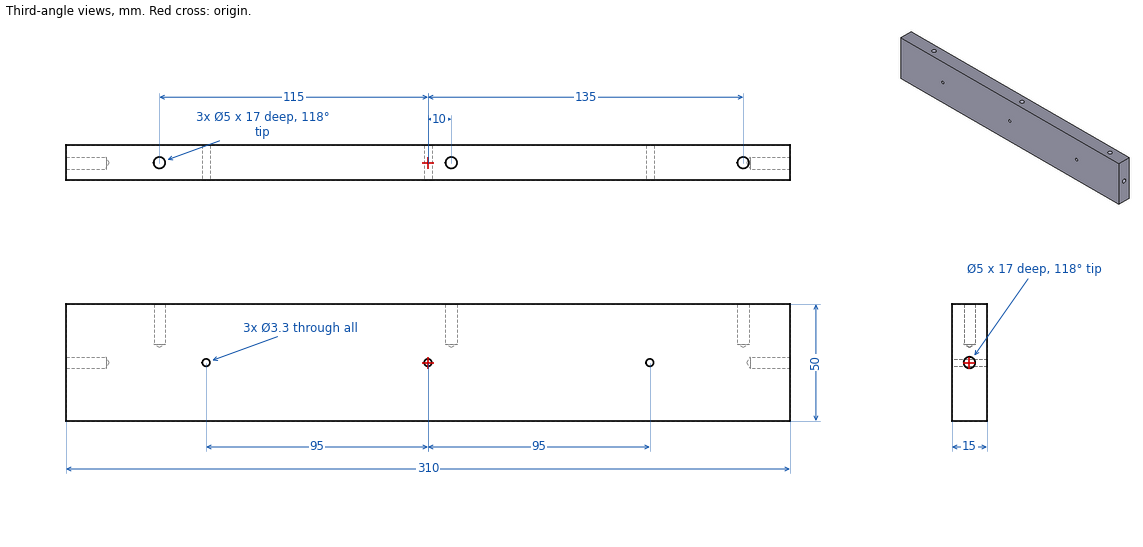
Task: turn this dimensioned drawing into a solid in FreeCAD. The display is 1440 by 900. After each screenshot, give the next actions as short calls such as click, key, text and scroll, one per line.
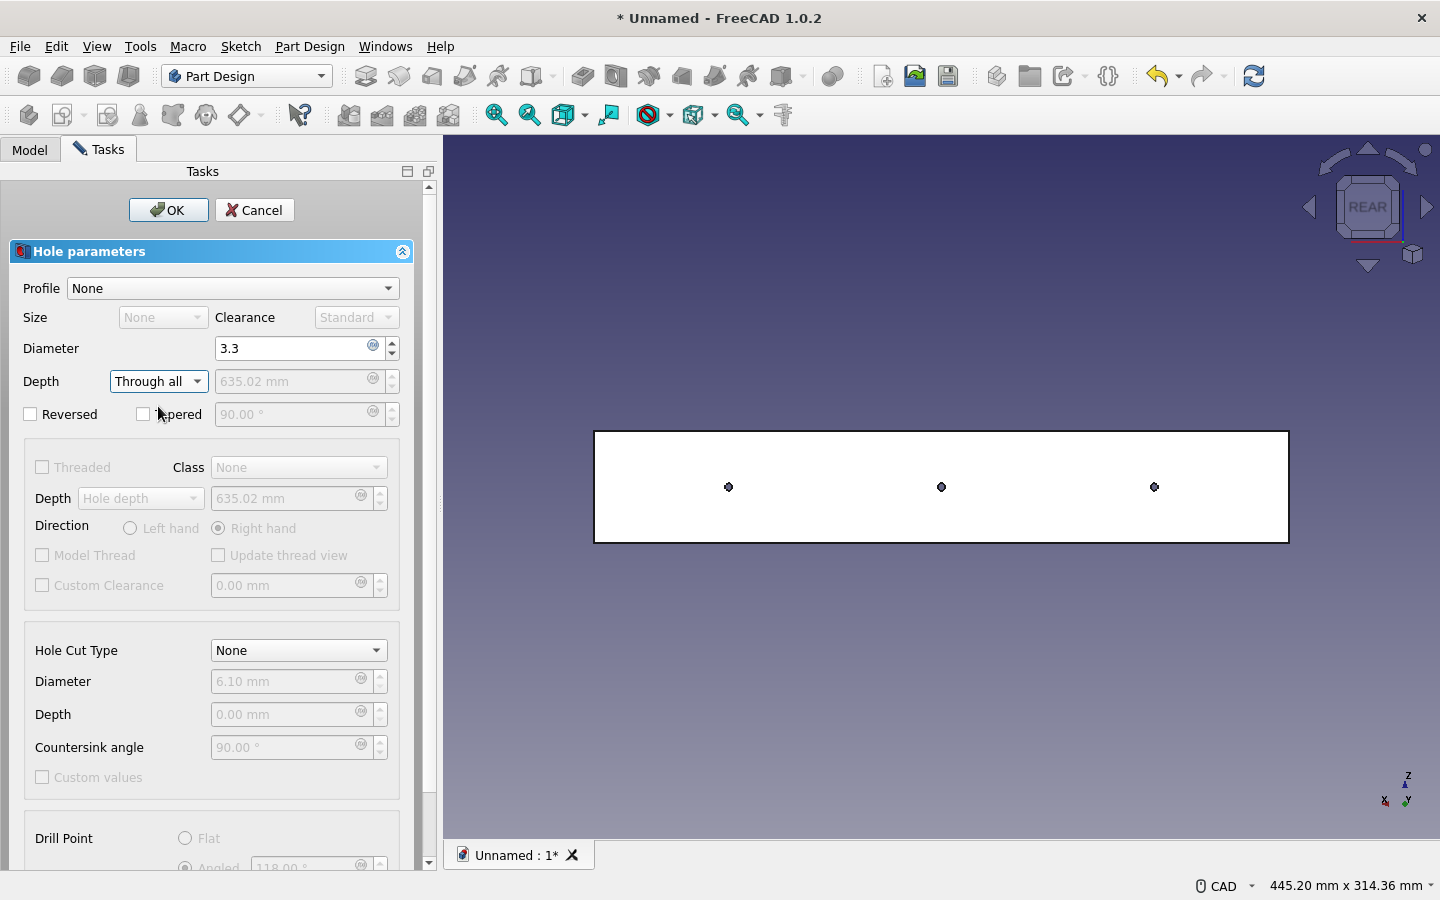
click(169, 210)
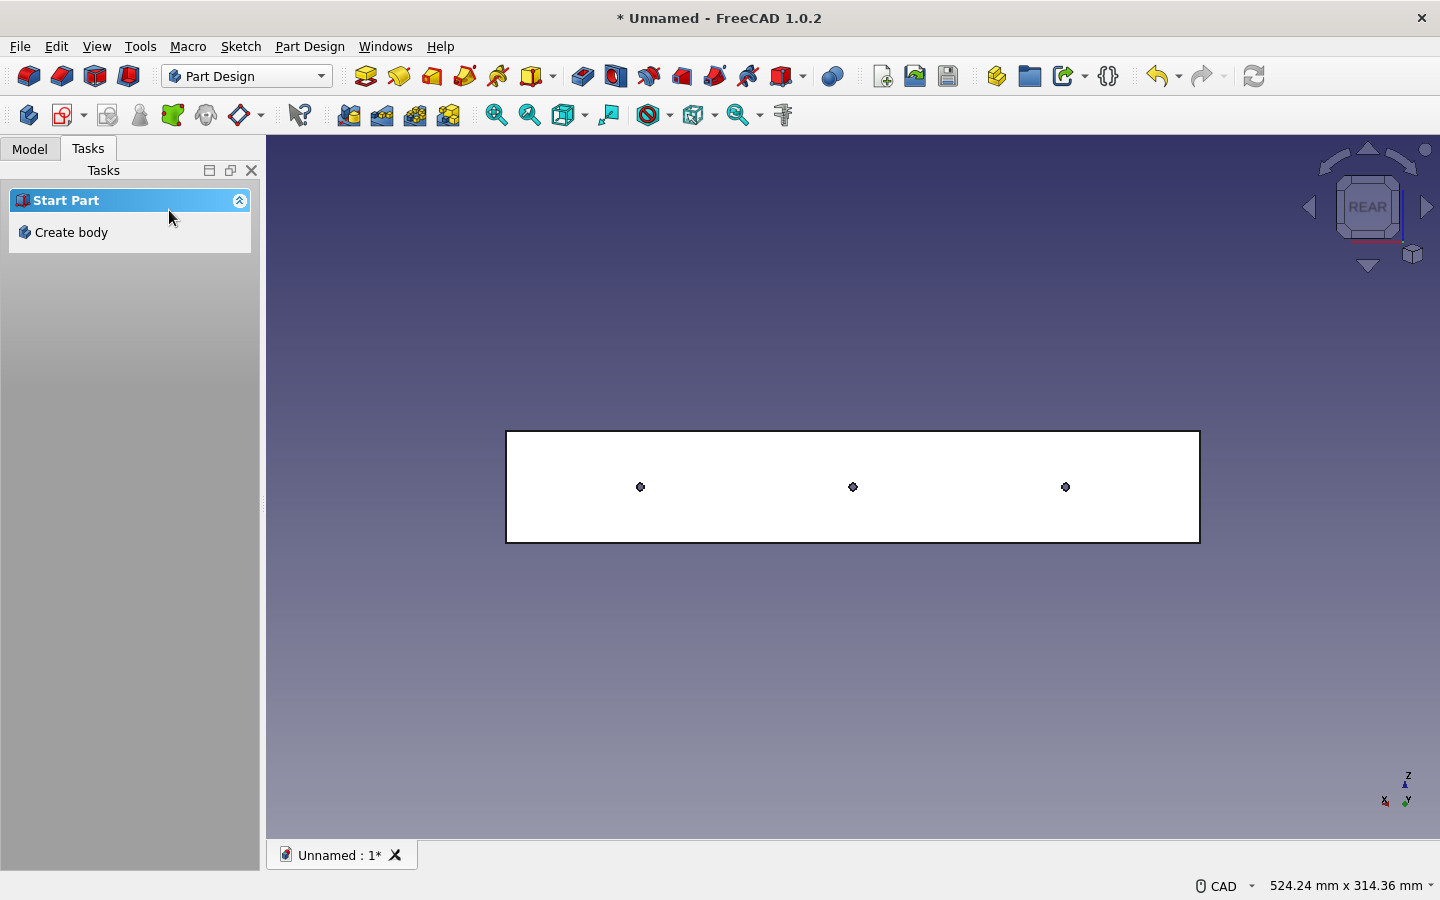
key(0)